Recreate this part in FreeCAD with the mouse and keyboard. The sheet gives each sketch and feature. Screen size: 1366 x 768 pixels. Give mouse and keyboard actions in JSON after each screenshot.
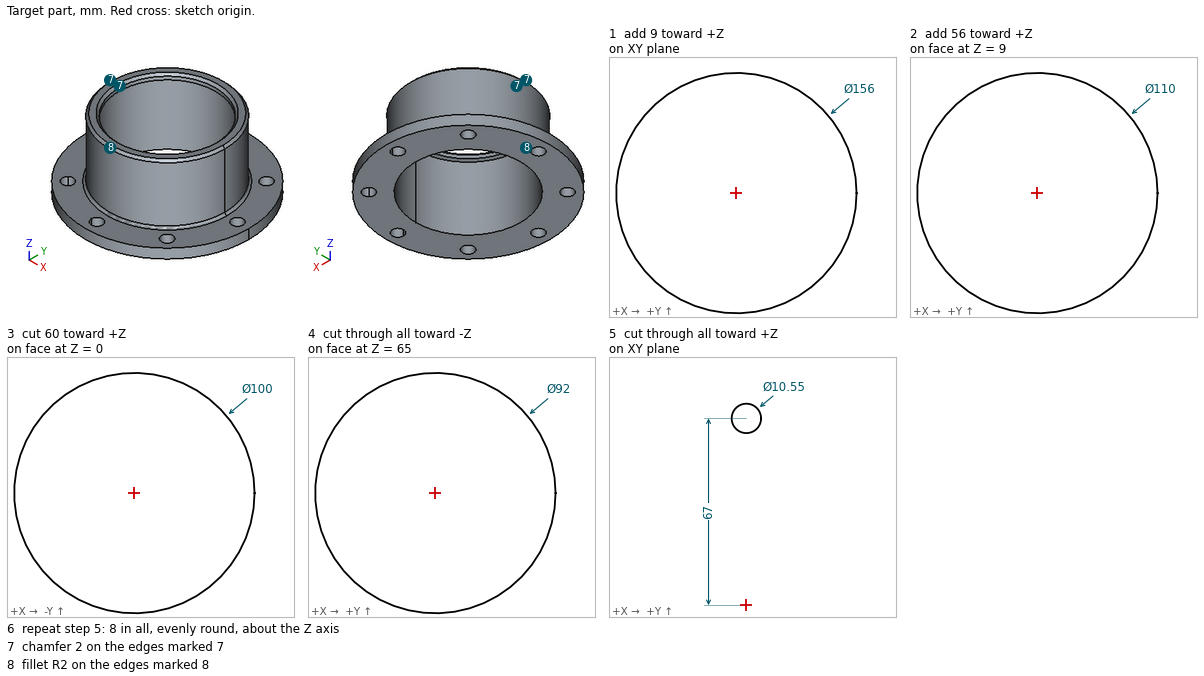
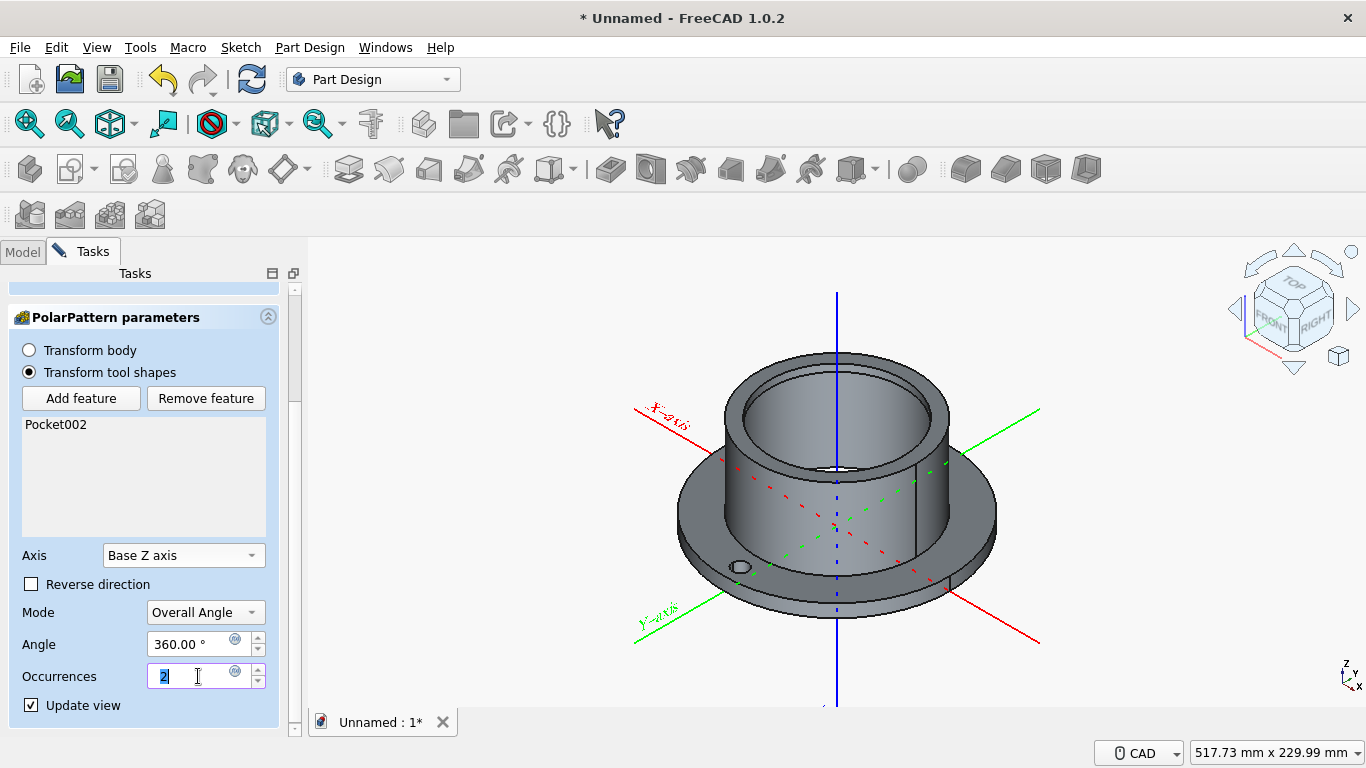
{"action": "type", "text": "8"}
{"action": "key", "text": "Tab"}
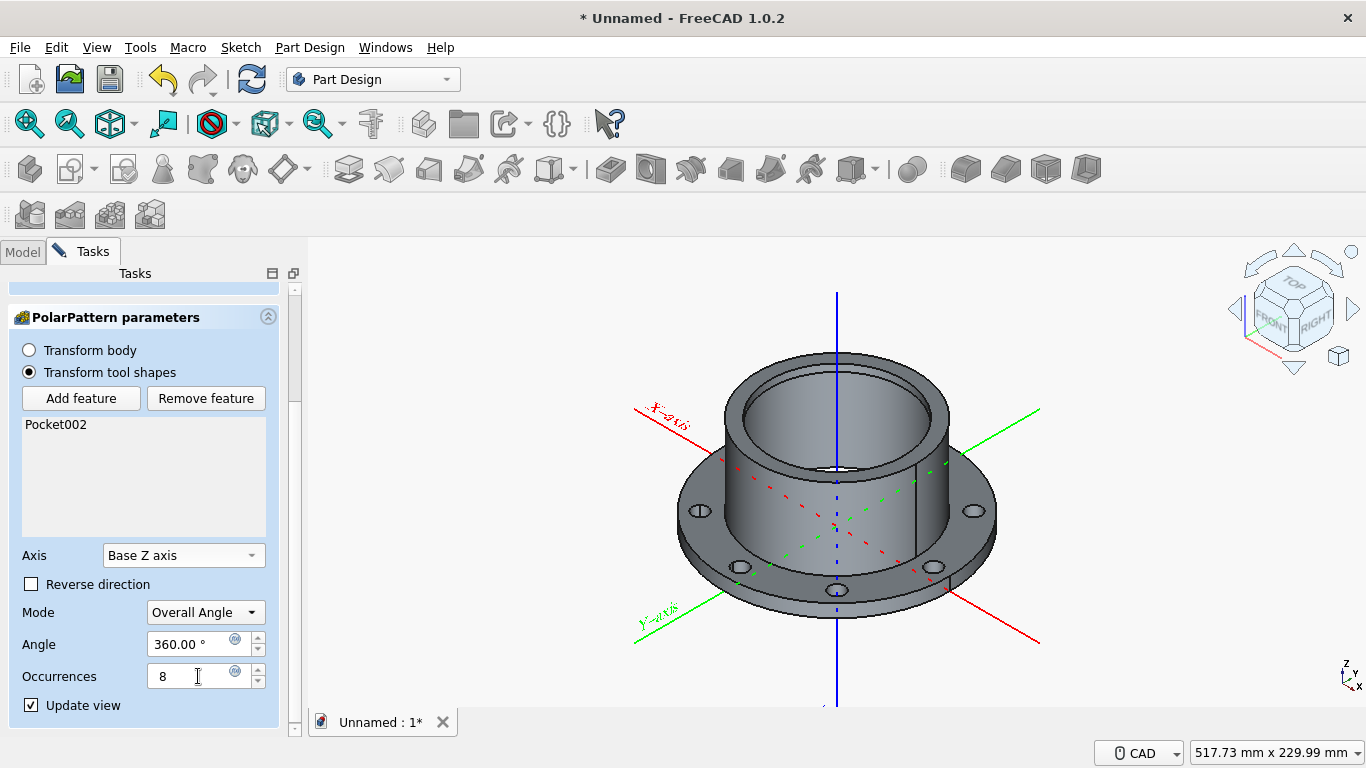
{"action": "scroll", "coordinate": [295, 510], "scroll_direction": "up", "scroll_amount": 4}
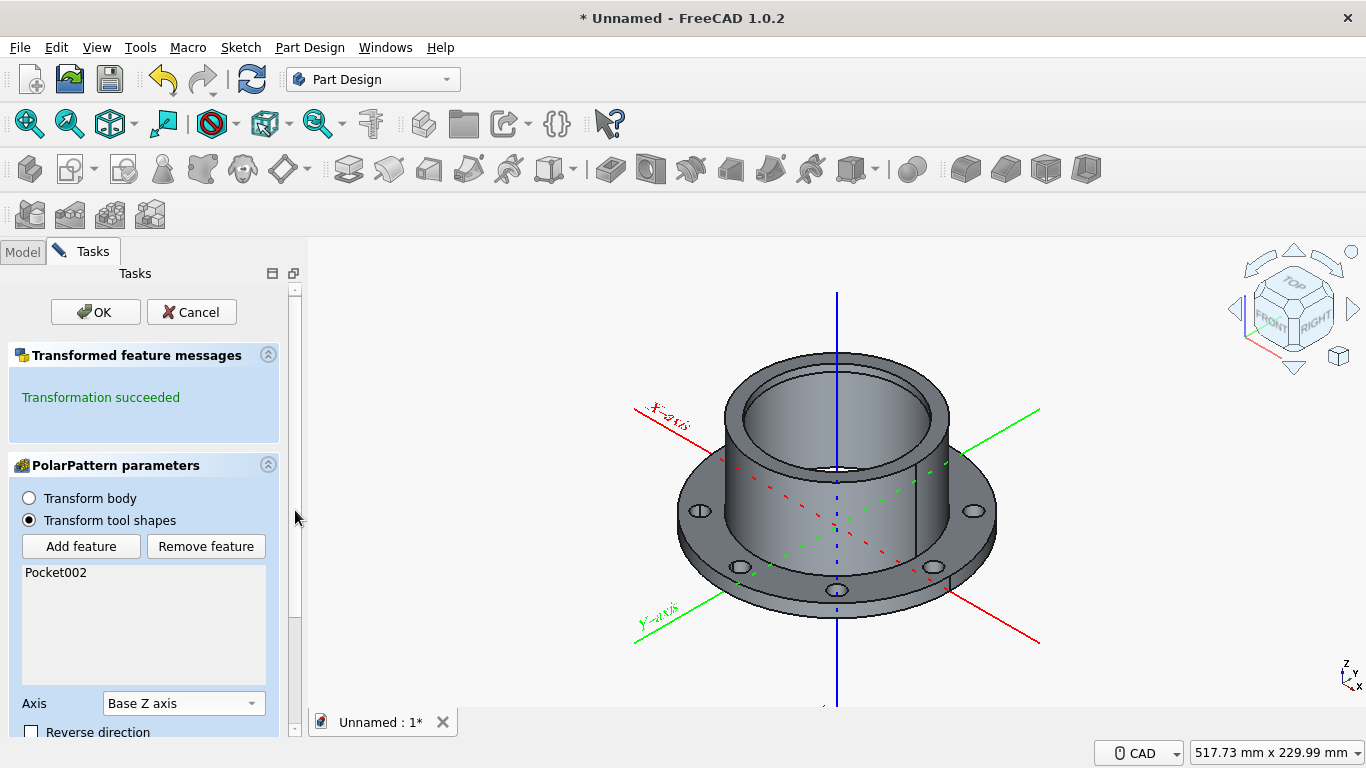
{"action": "left_click", "coordinate": [96, 312]}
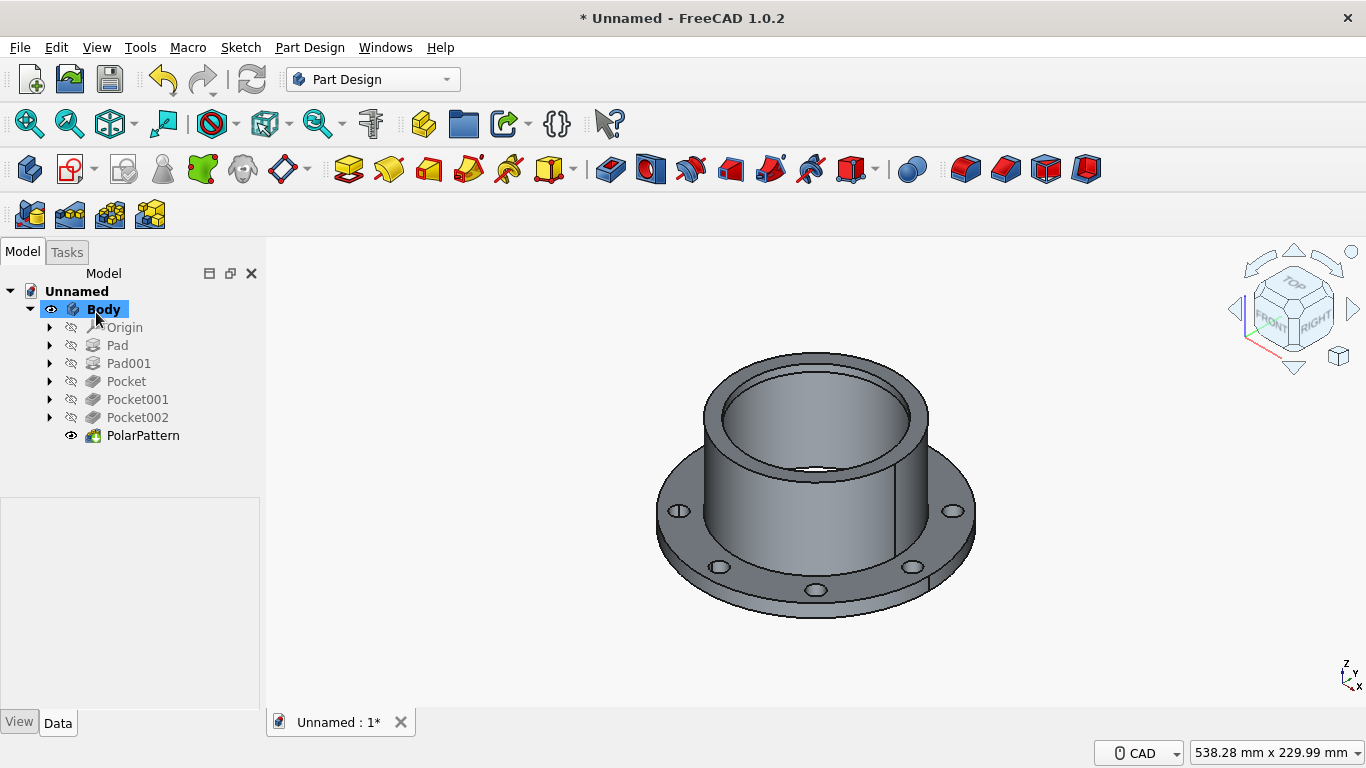
{"action": "left_click", "coordinate": [750, 378]}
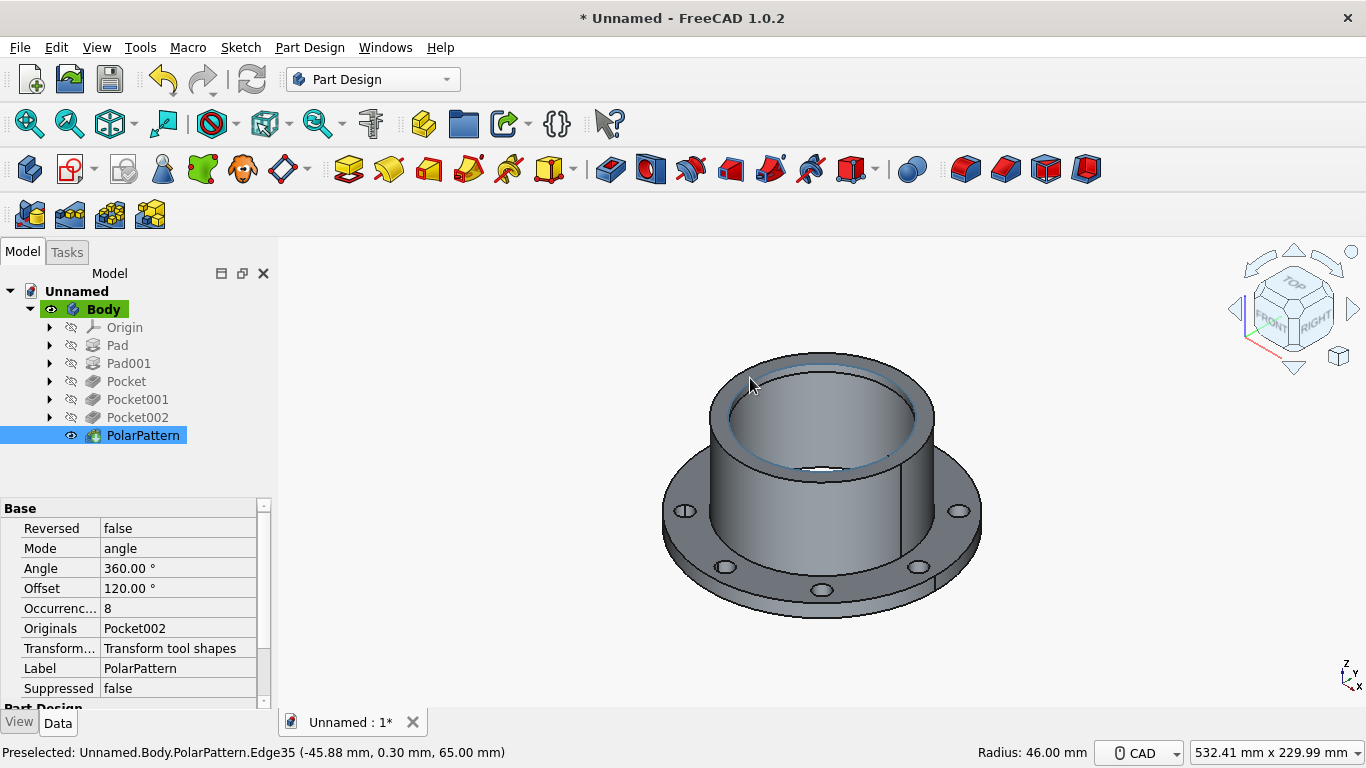
{"action": "left_click", "coordinate": [722, 446], "text": "ctrl"}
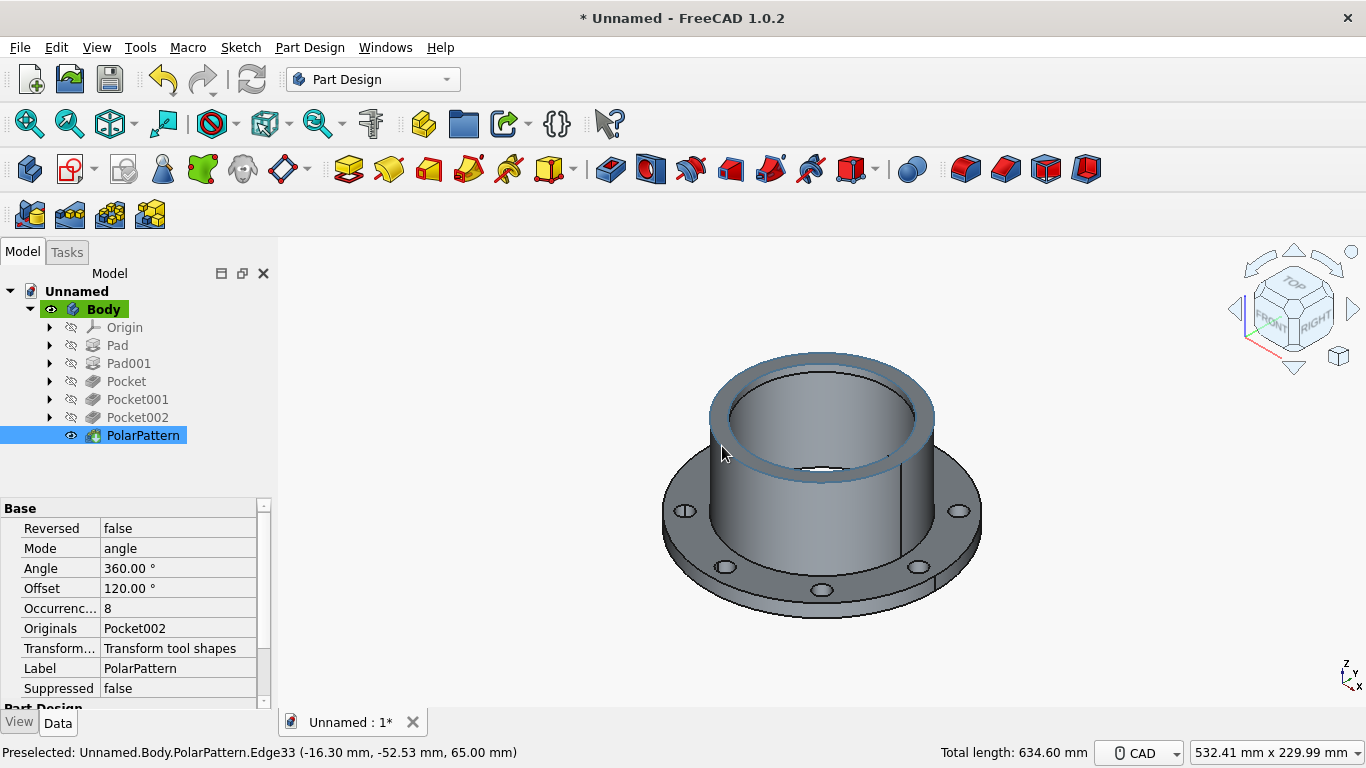
{"action": "left_click", "coordinate": [1006, 170]}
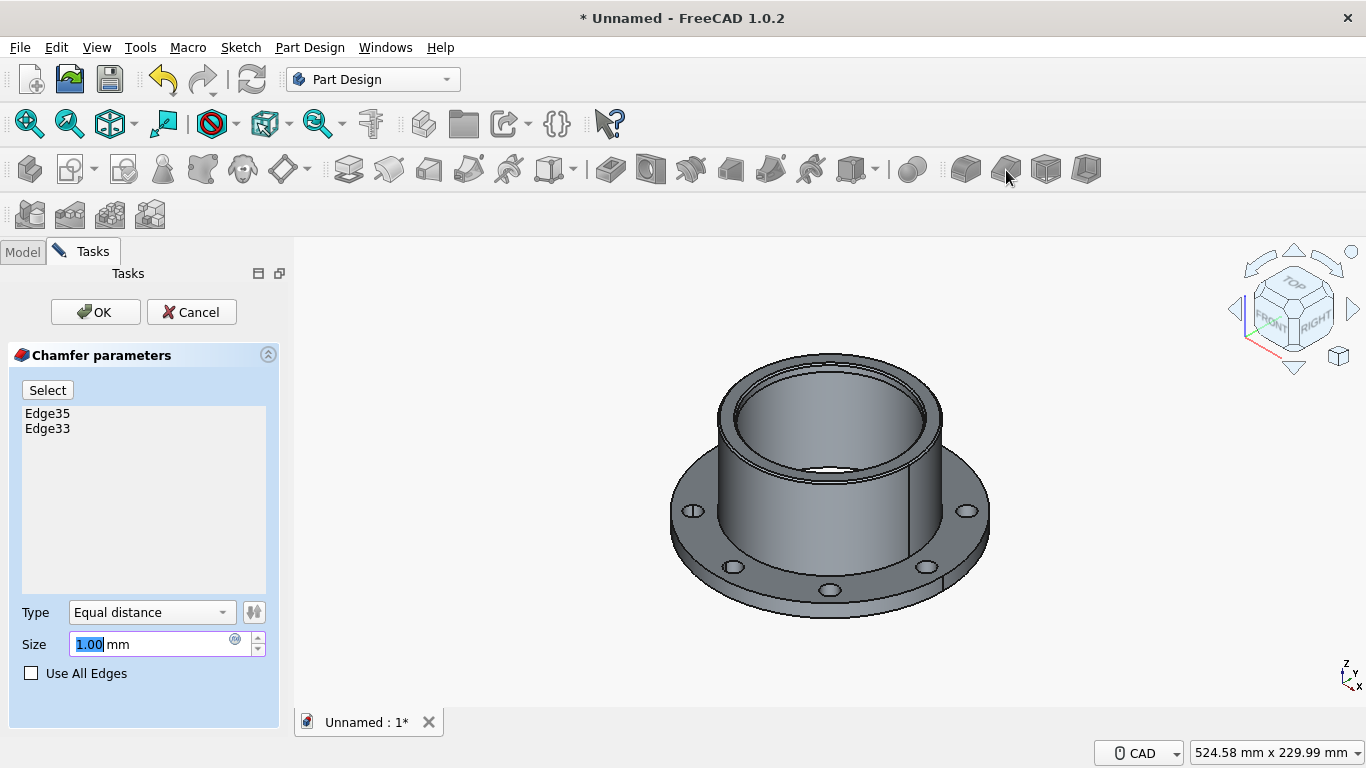
{"action": "type", "text": "2"}
{"action": "key", "text": "Tab"}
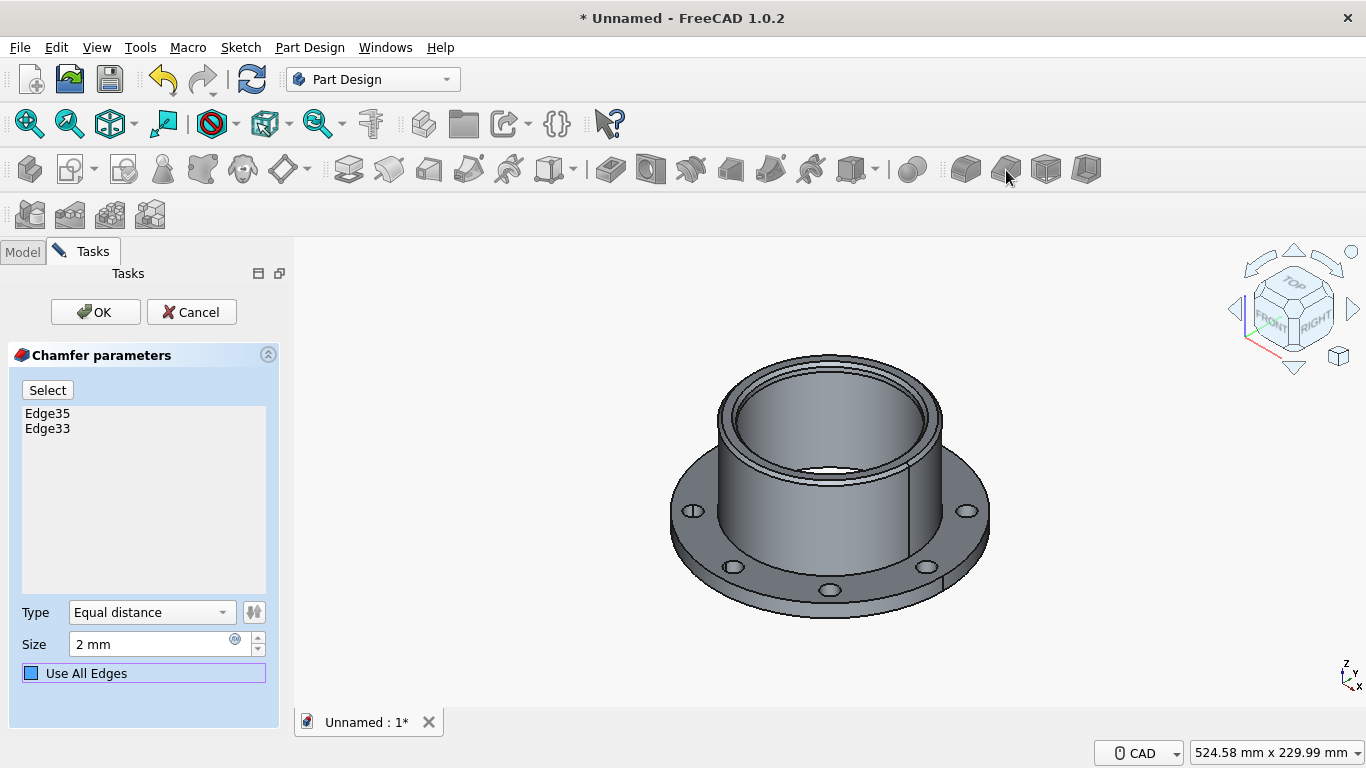
{"action": "left_click", "coordinate": [96, 312]}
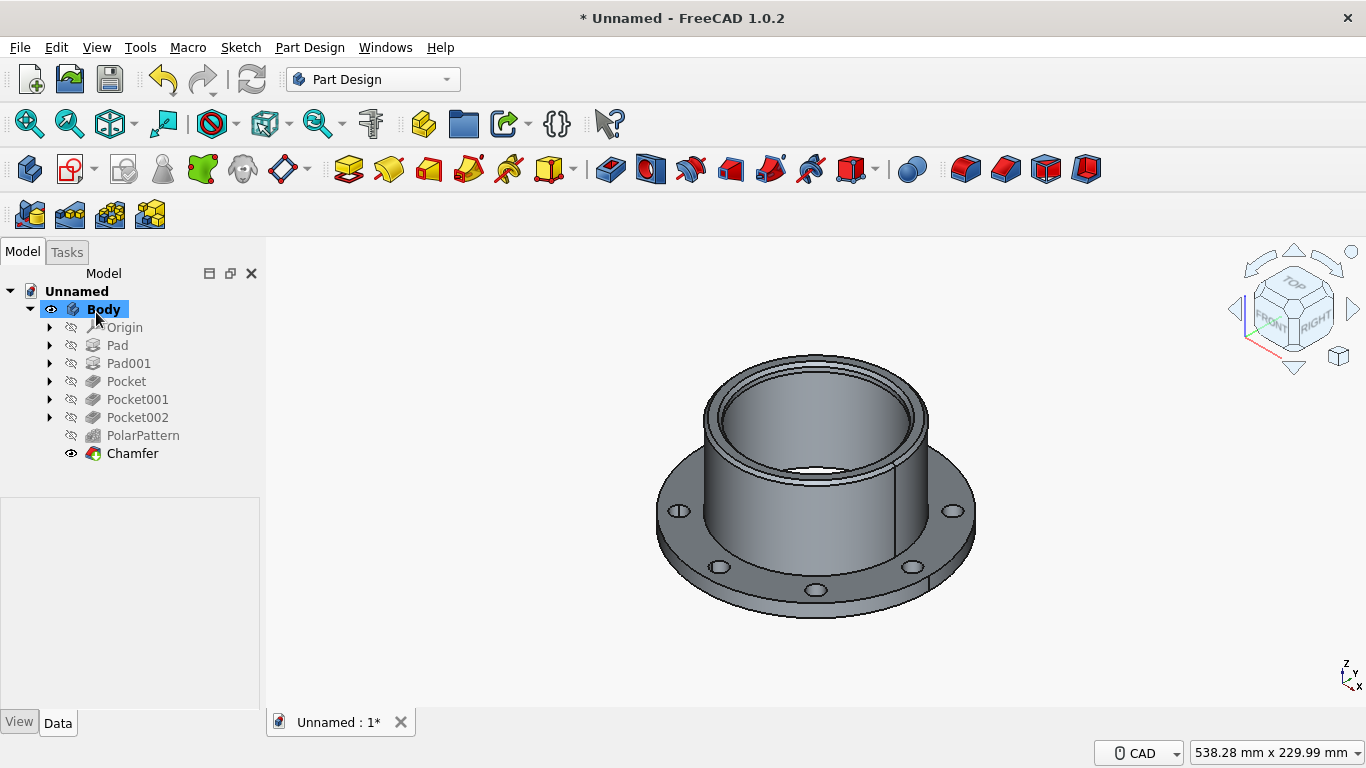
{"action": "key", "text": "2"}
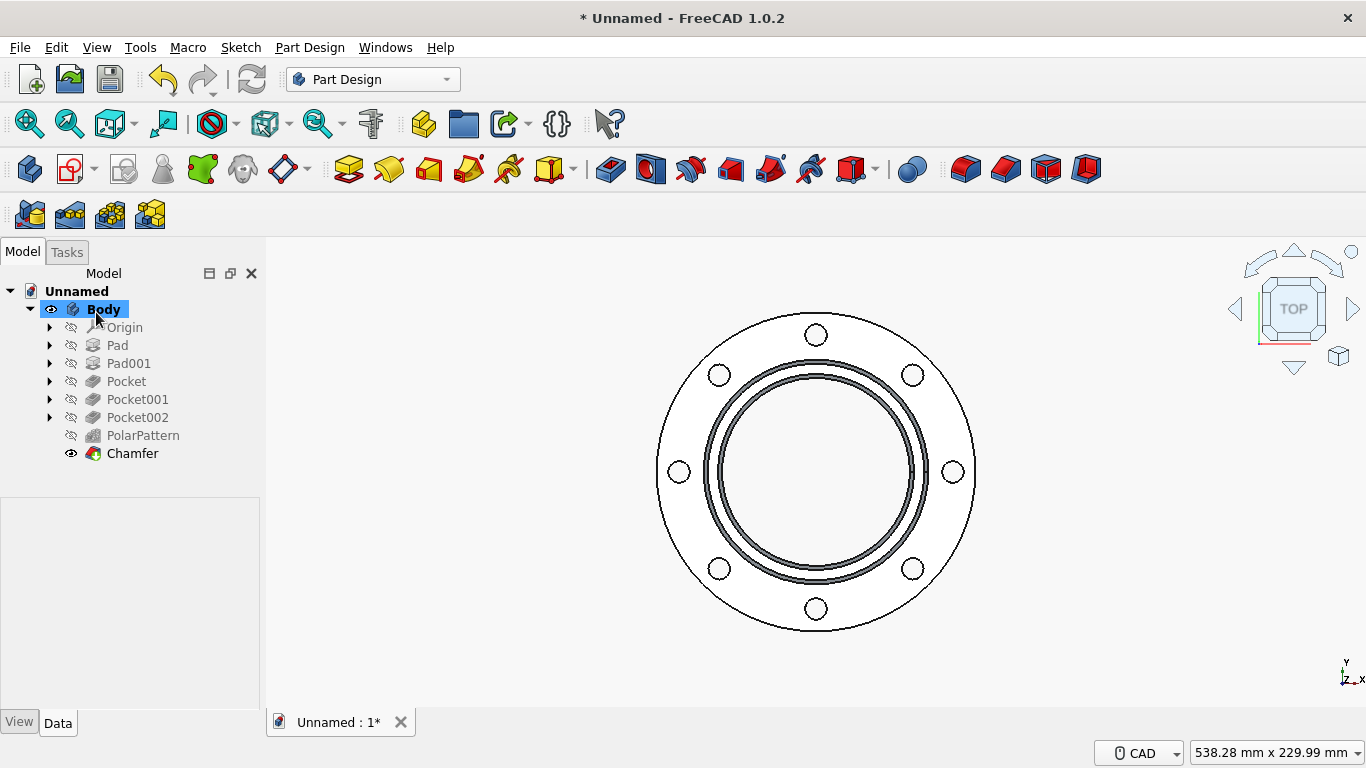
{"action": "key", "text": "0"}